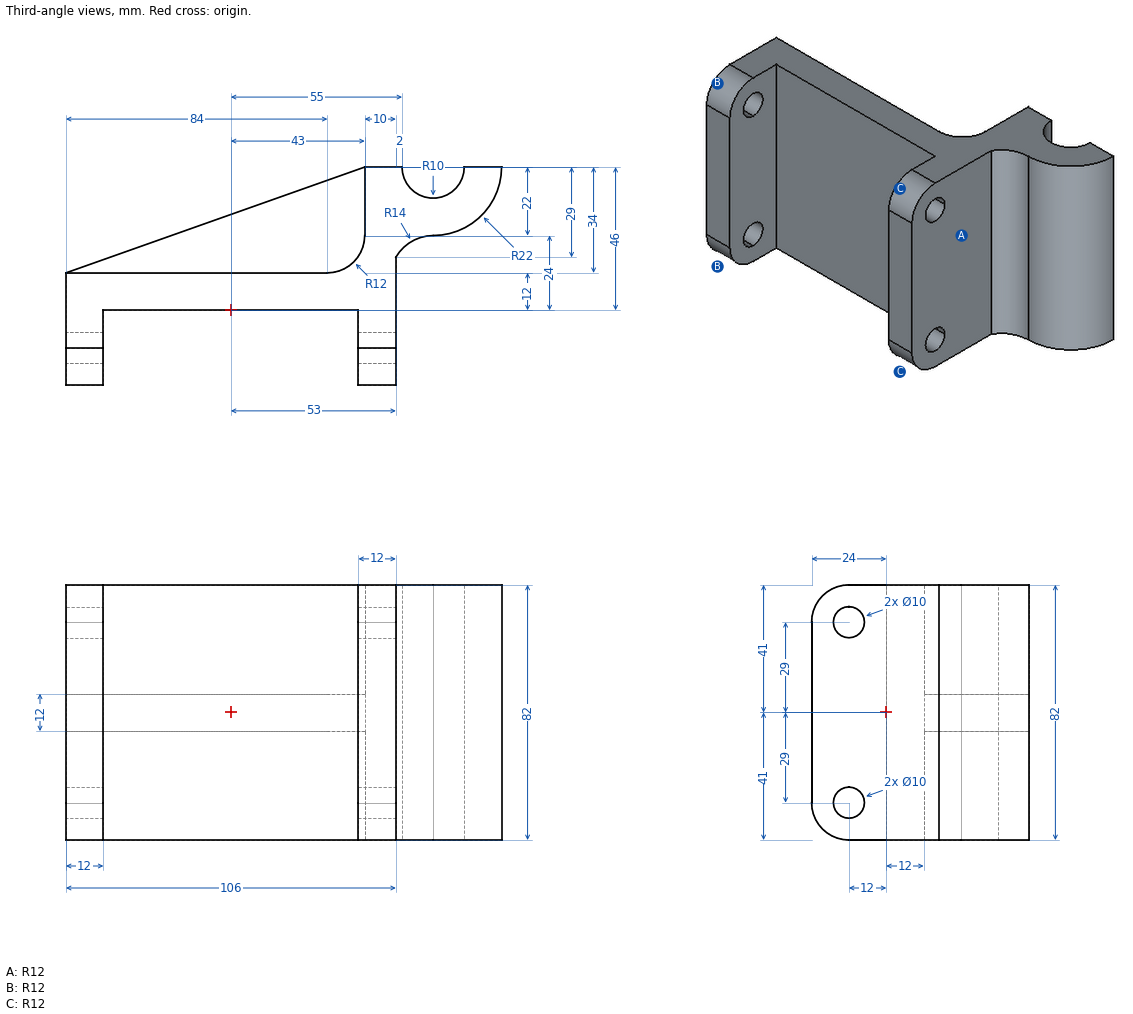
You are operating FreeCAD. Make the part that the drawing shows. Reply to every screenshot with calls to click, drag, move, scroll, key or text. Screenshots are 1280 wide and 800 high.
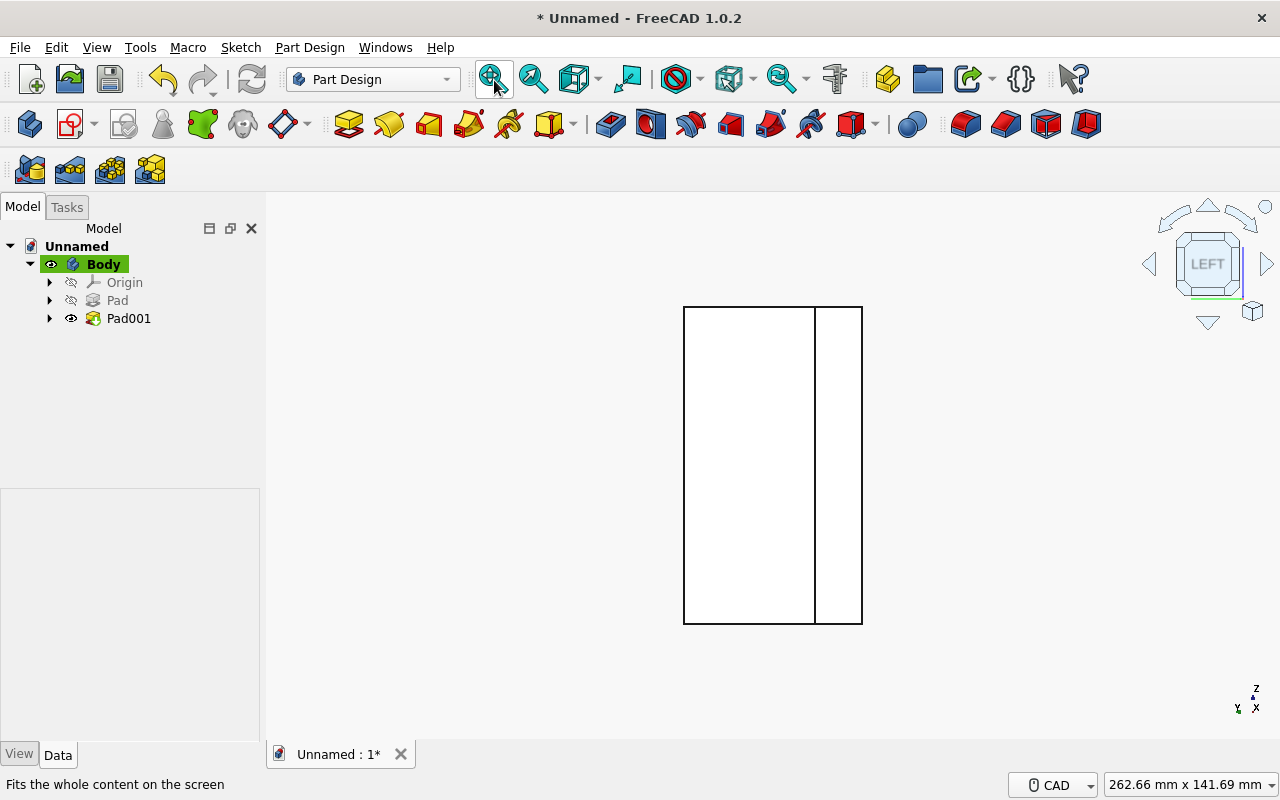
key(v)
key(3)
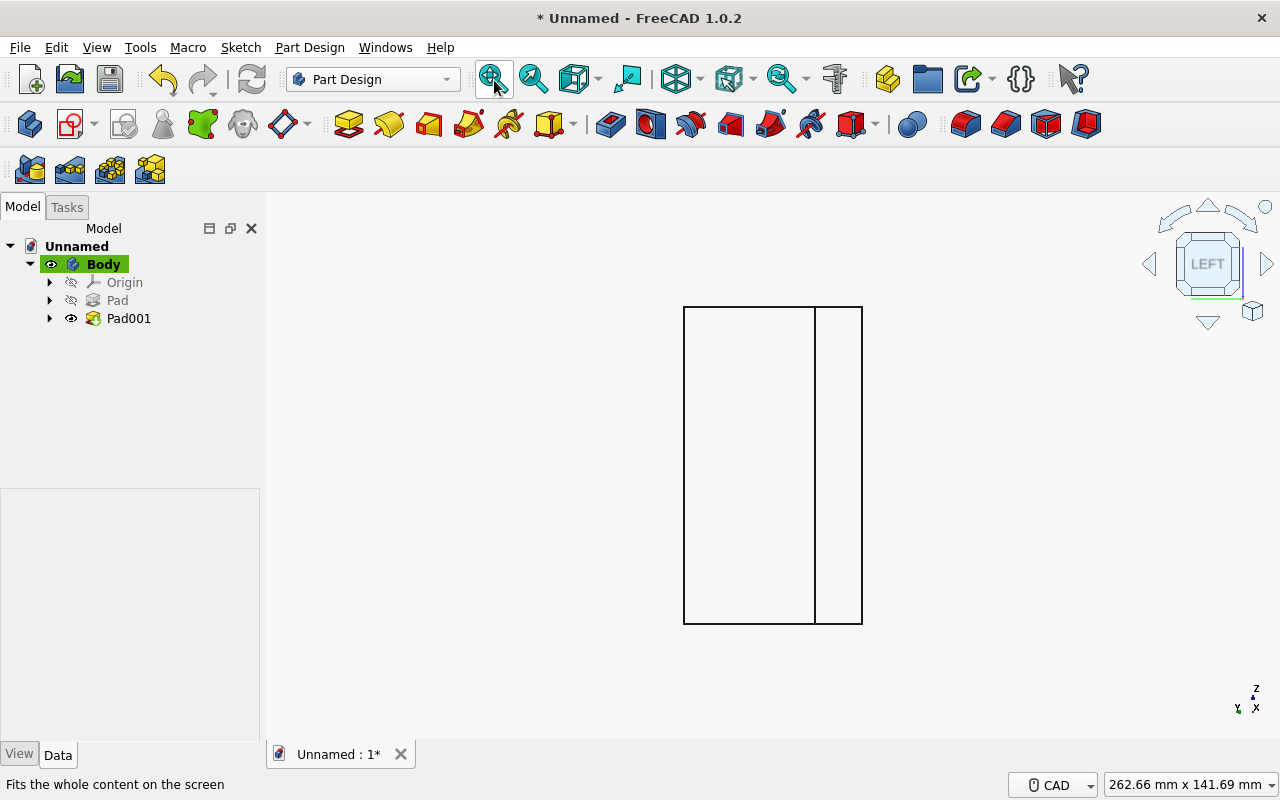
key(0)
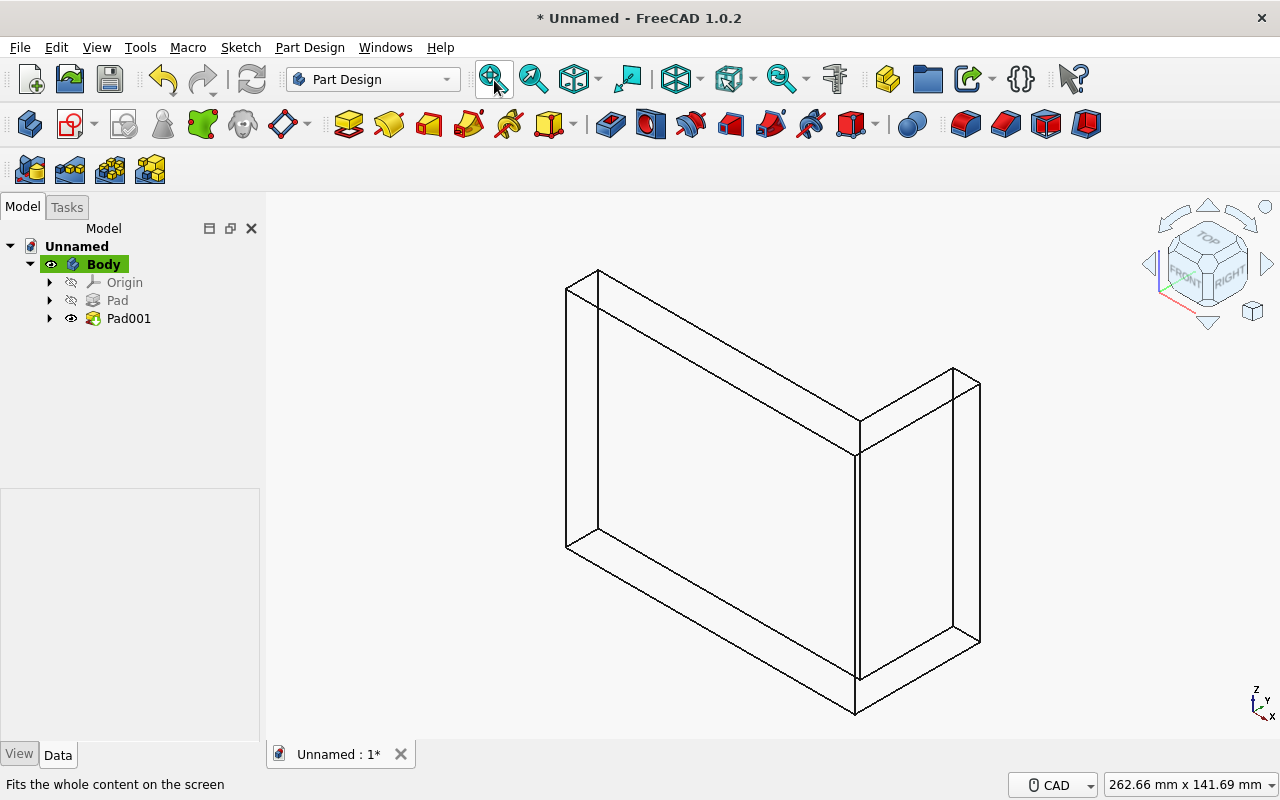
click(860, 428)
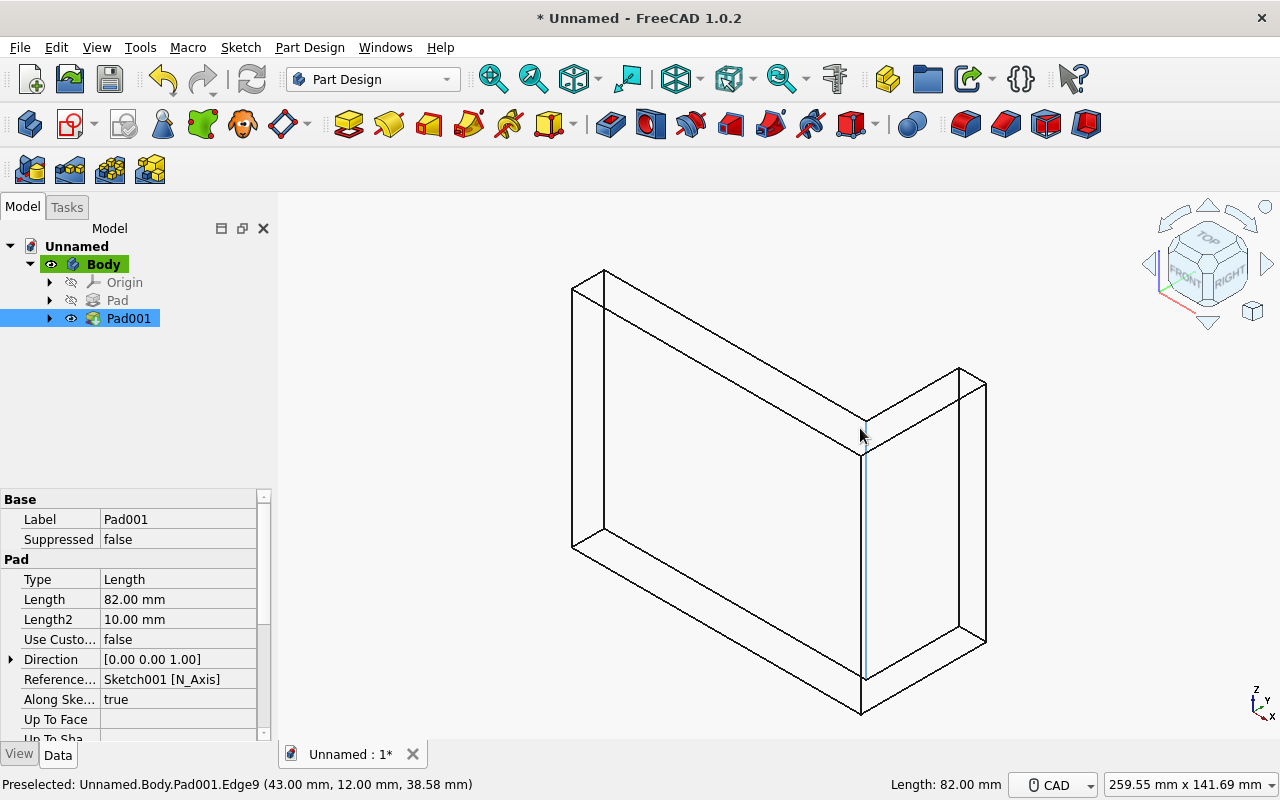
key(v)
key(1)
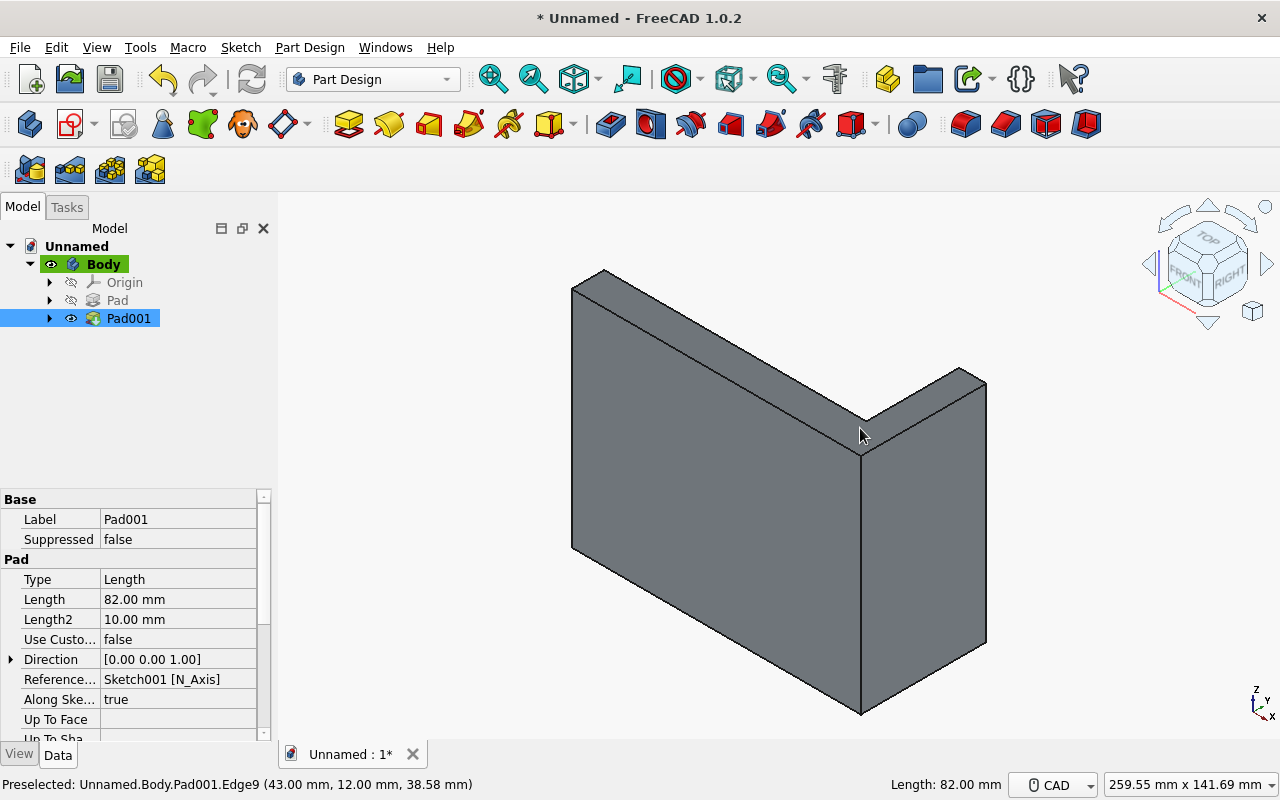
click(966, 124)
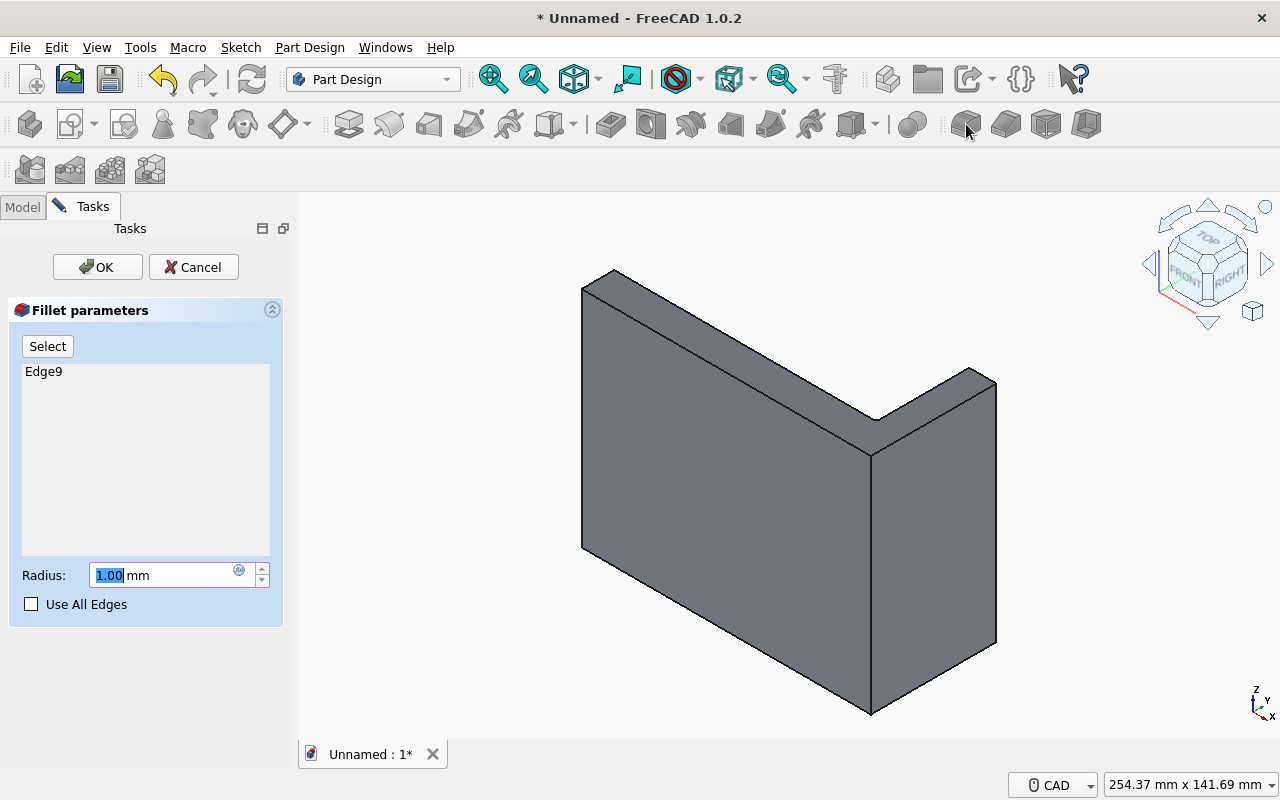
text(12)
key(Tab)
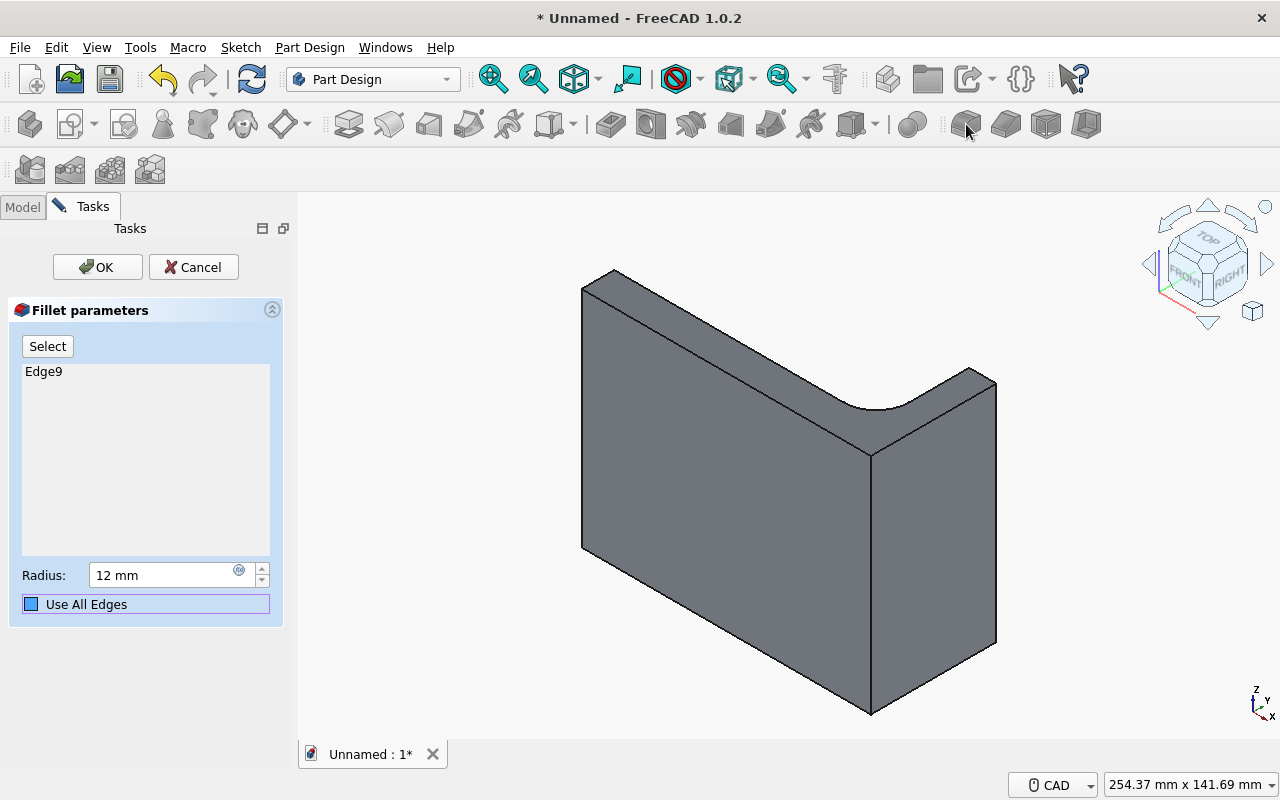
click(98, 267)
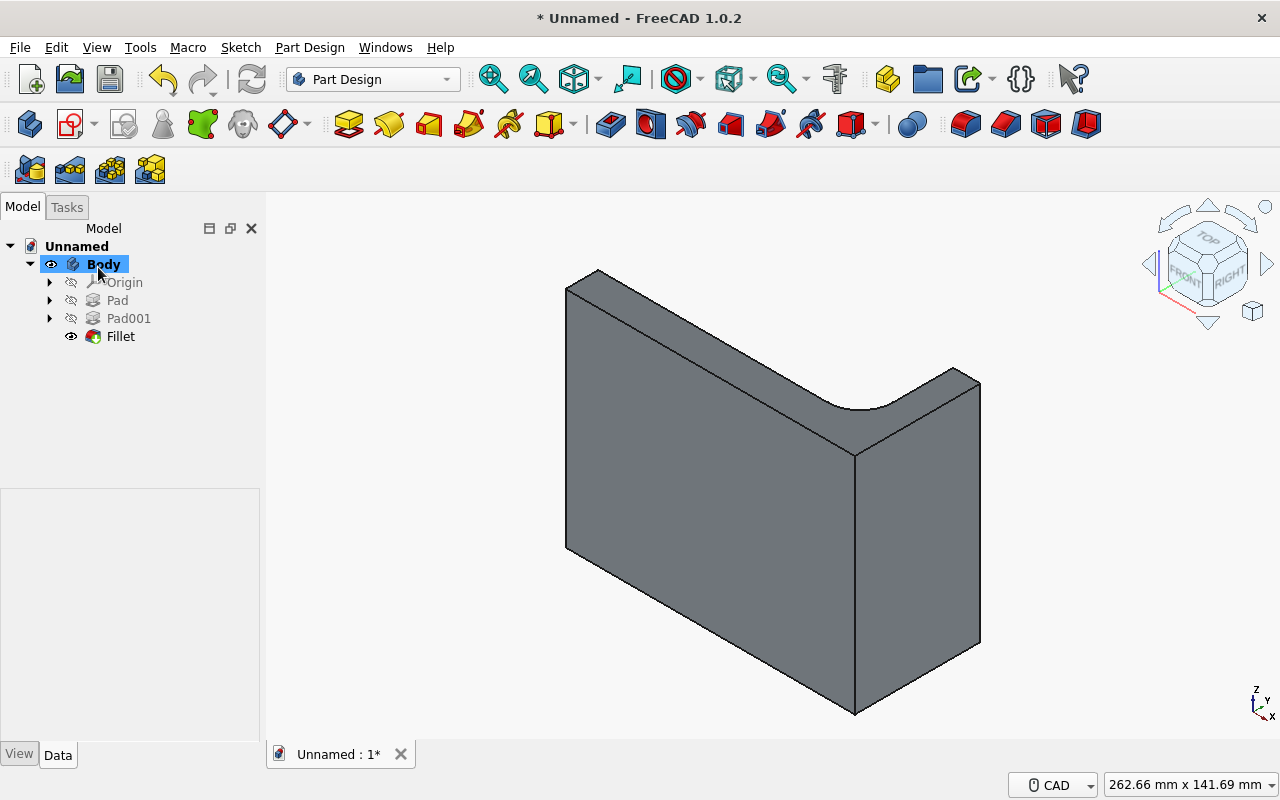
key(6)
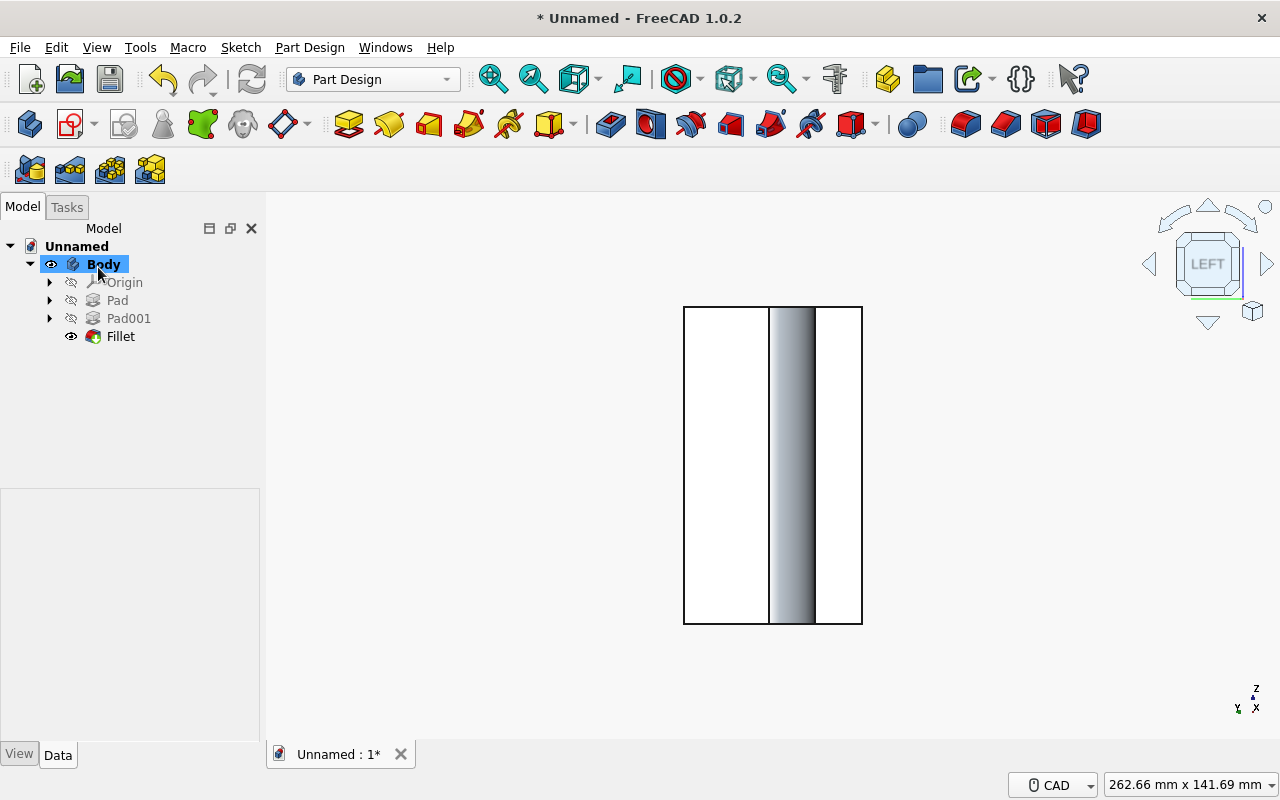
click(839, 374)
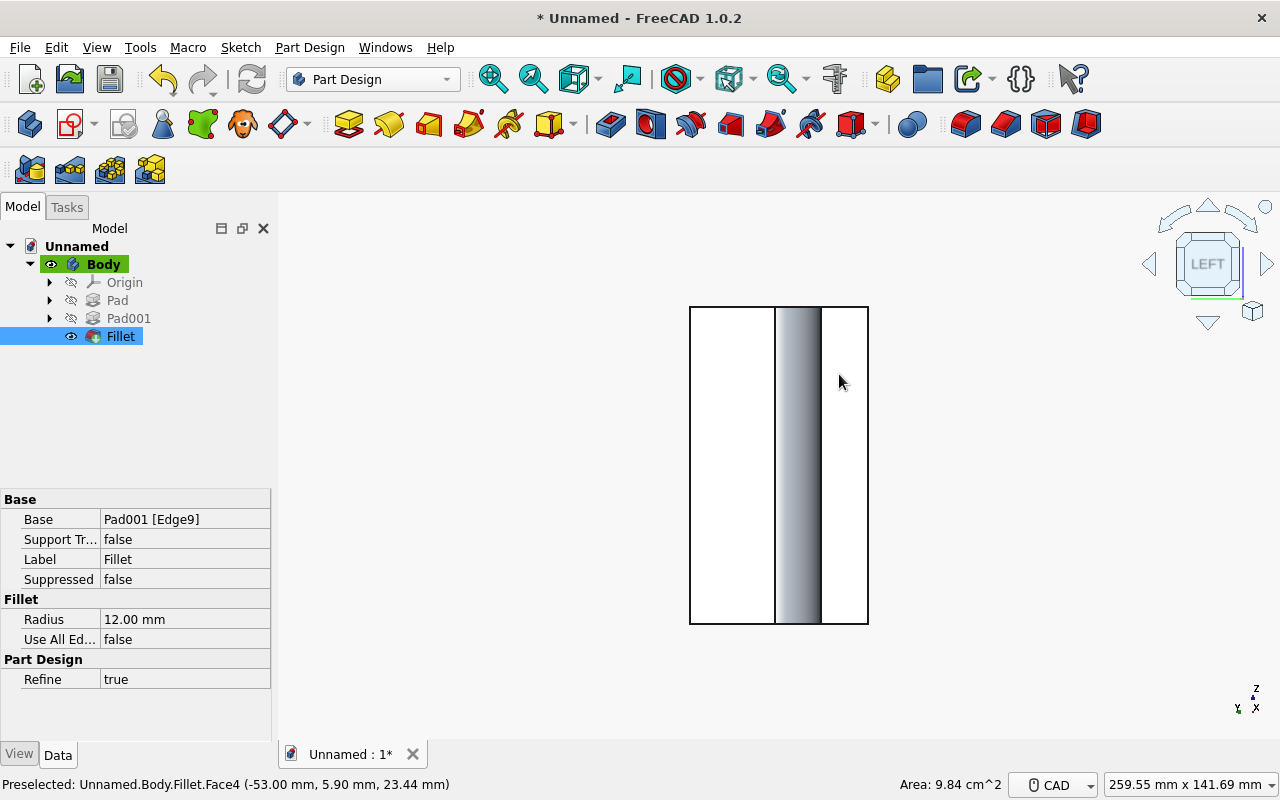
click(70, 124)